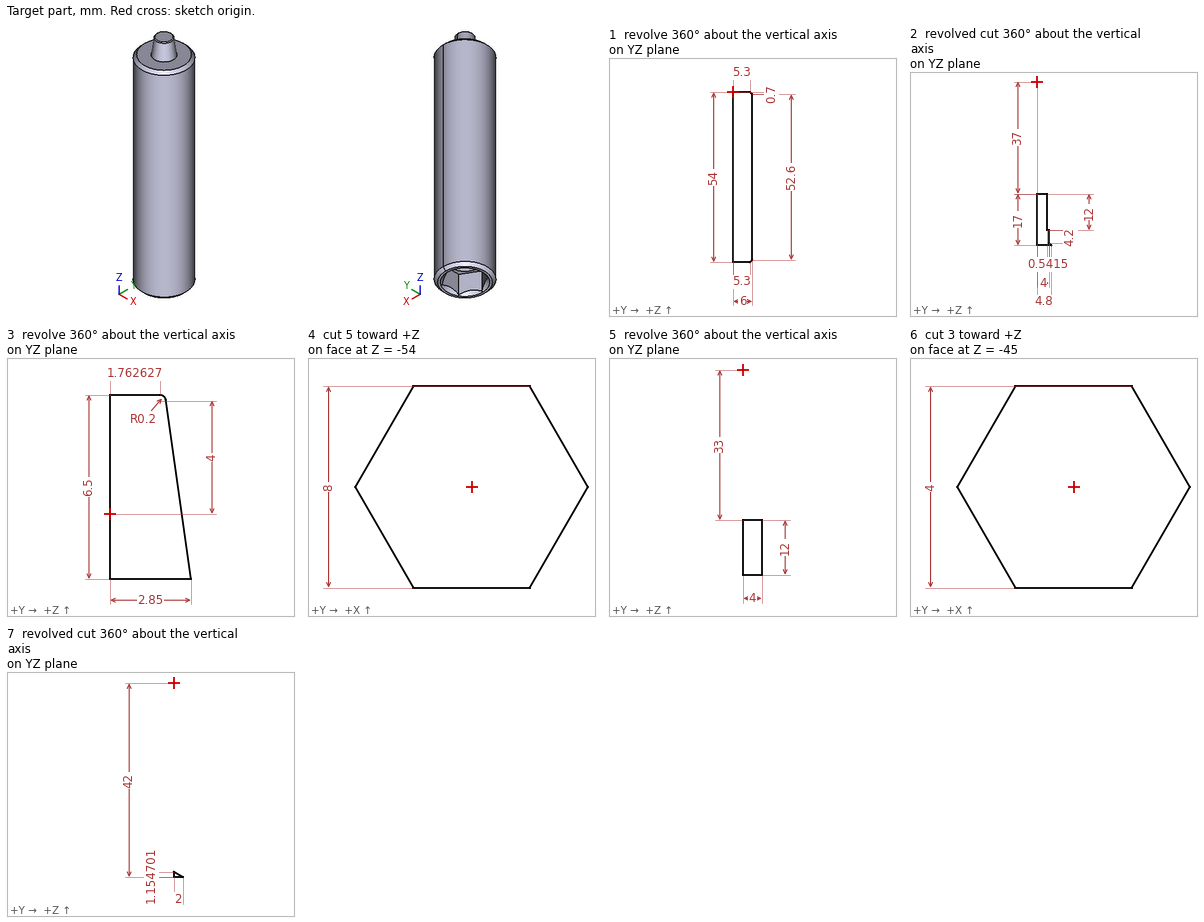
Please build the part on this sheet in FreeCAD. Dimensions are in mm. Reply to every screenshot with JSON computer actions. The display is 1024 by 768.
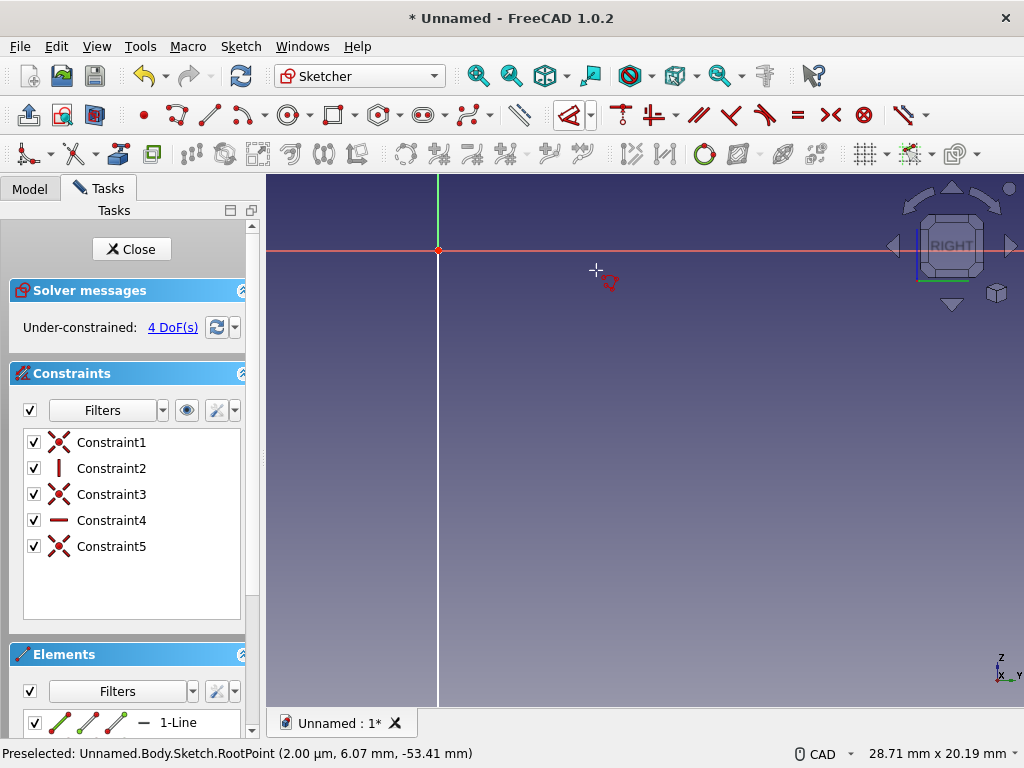
{"action": "left_click", "coordinate": [597, 269]}
{"action": "left_click", "coordinate": [578, 260]}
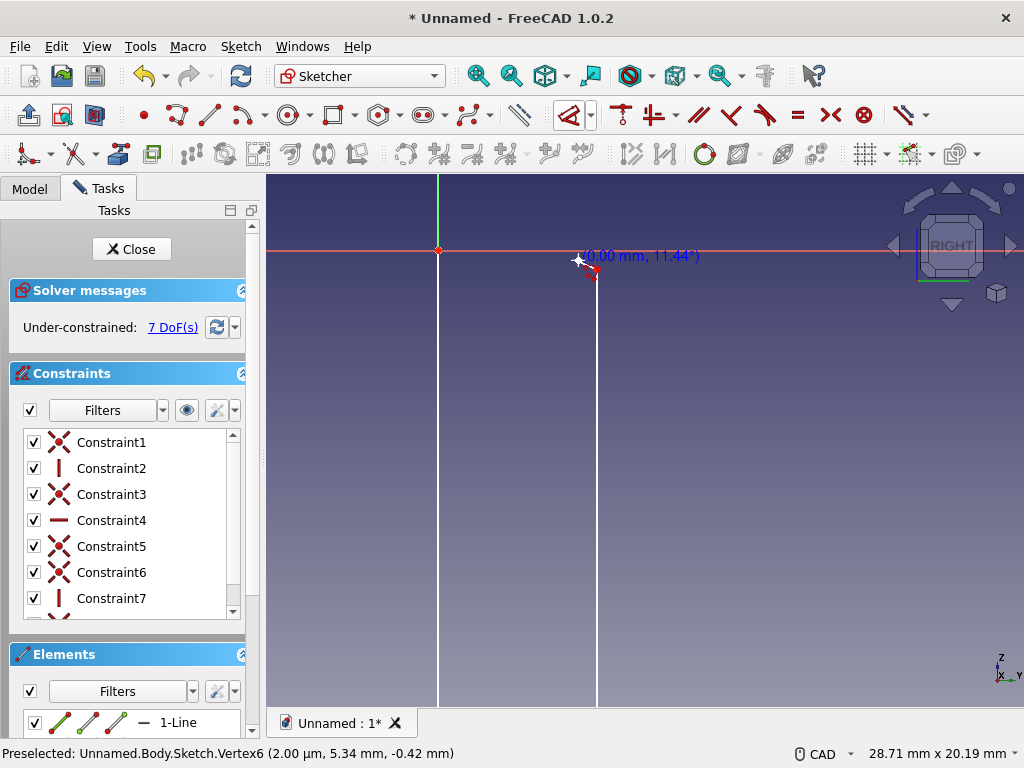
{"action": "scroll", "coordinate": [596, 269], "scroll_direction": "down", "scroll_amount": 7}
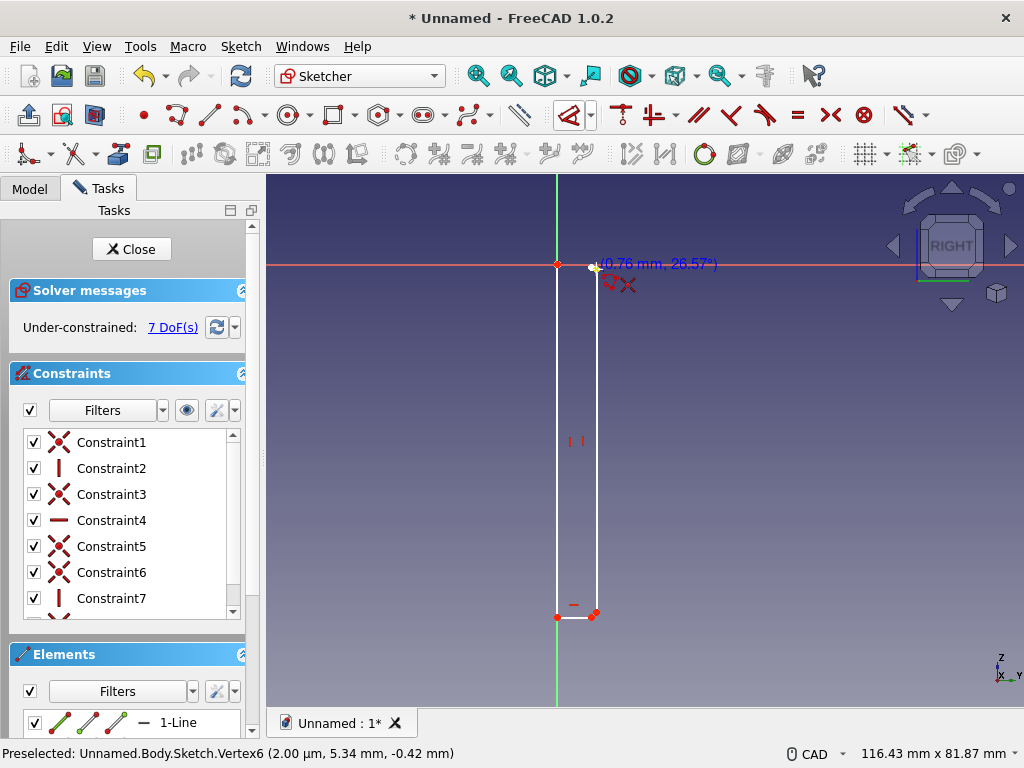
{"action": "left_click", "coordinate": [557, 265]}
{"action": "key", "text": "Escape"}
{"action": "key", "text": "Escape"}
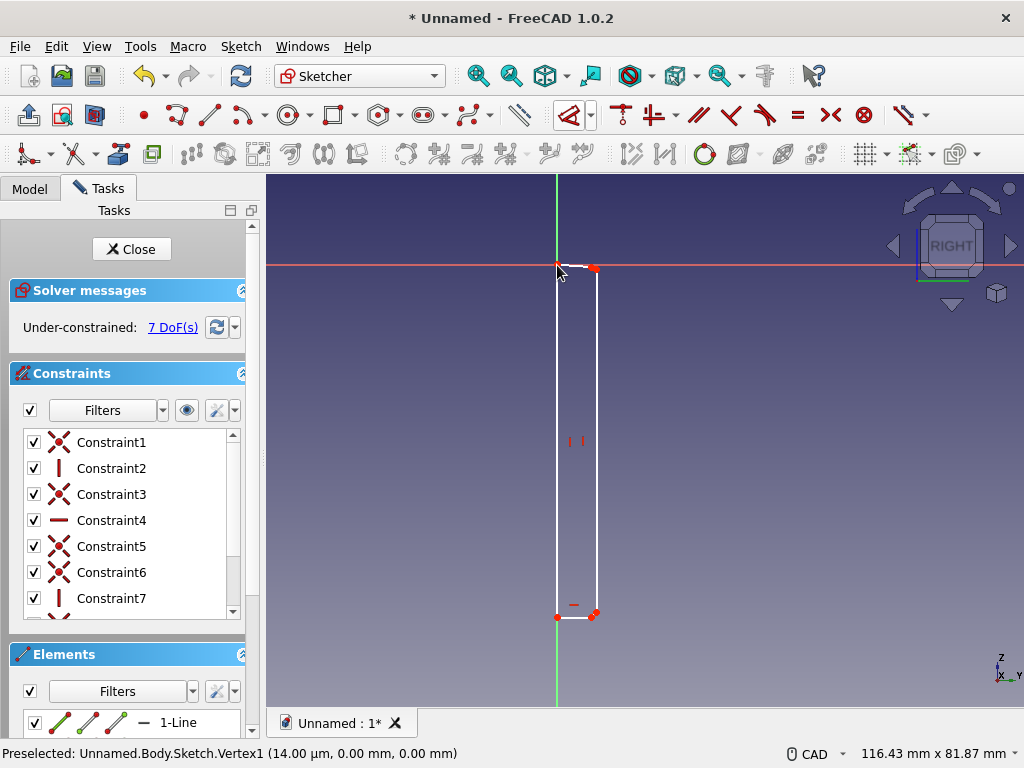
{"action": "scroll", "coordinate": [582, 266], "scroll_direction": "up", "scroll_amount": 2}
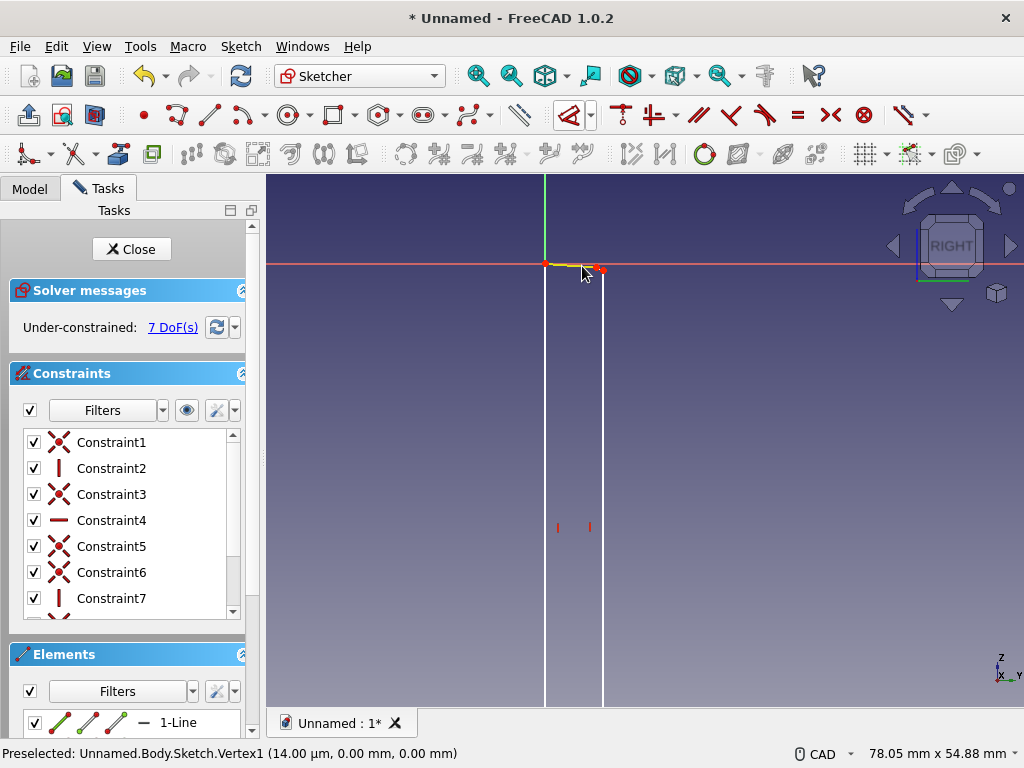
{"action": "left_click", "coordinate": [581, 267]}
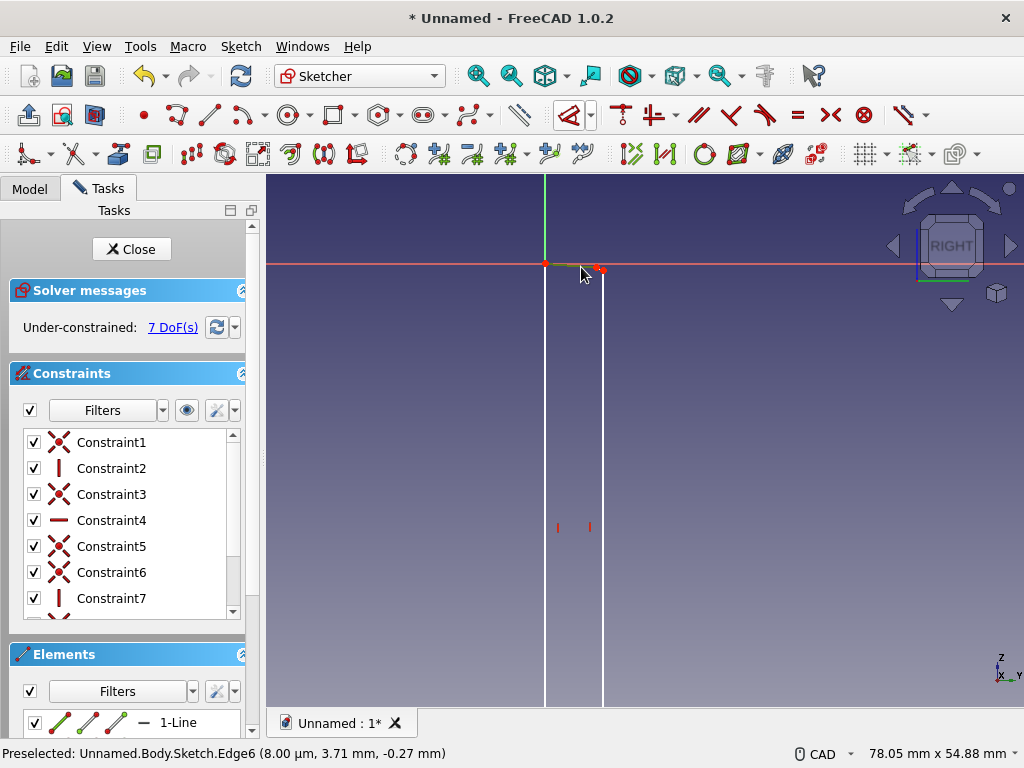
{"action": "key", "text": "h"}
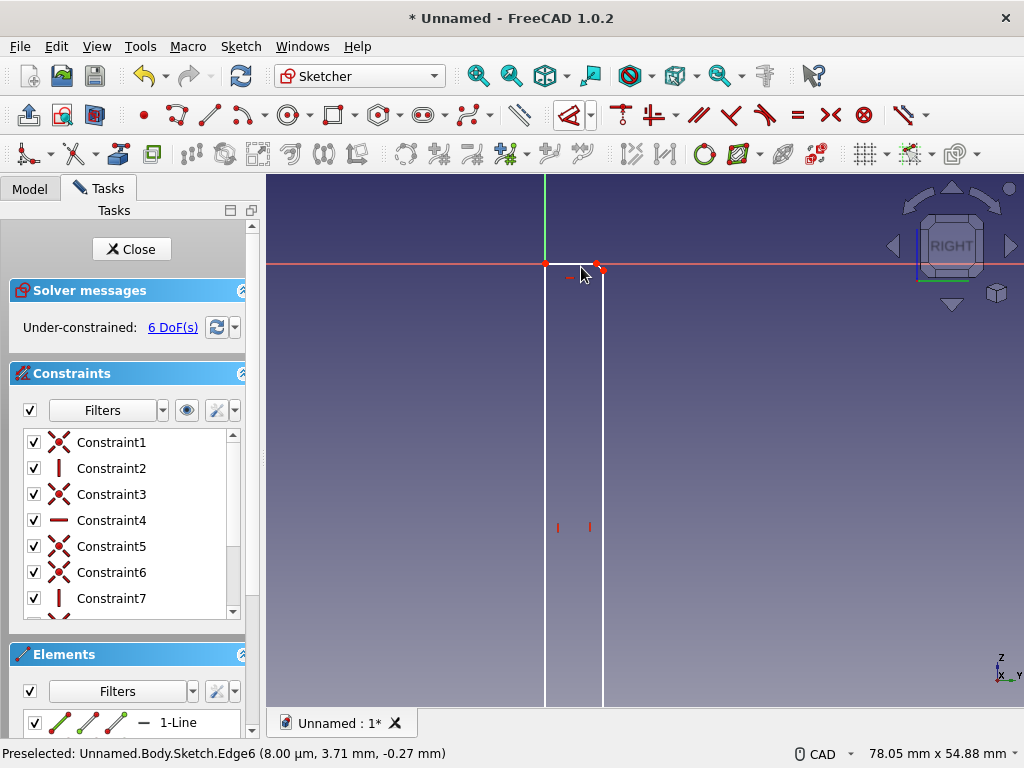
{"action": "left_click", "coordinate": [568, 116]}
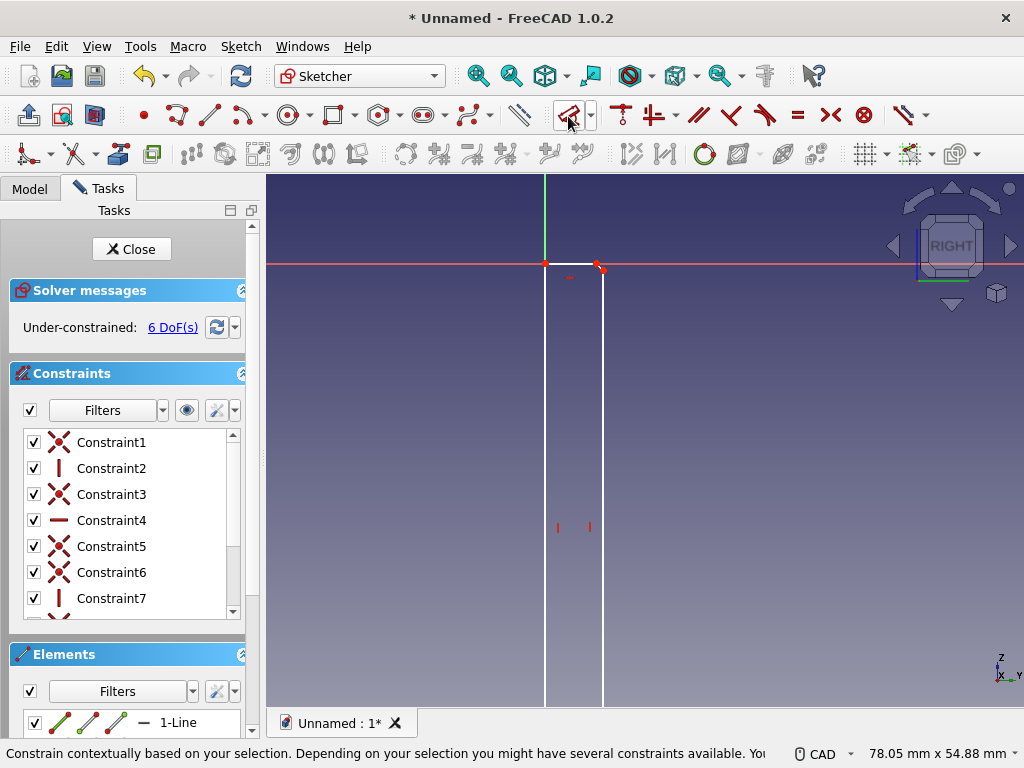
{"action": "left_click", "coordinate": [545, 422]}
{"action": "left_click", "coordinate": [511, 471]}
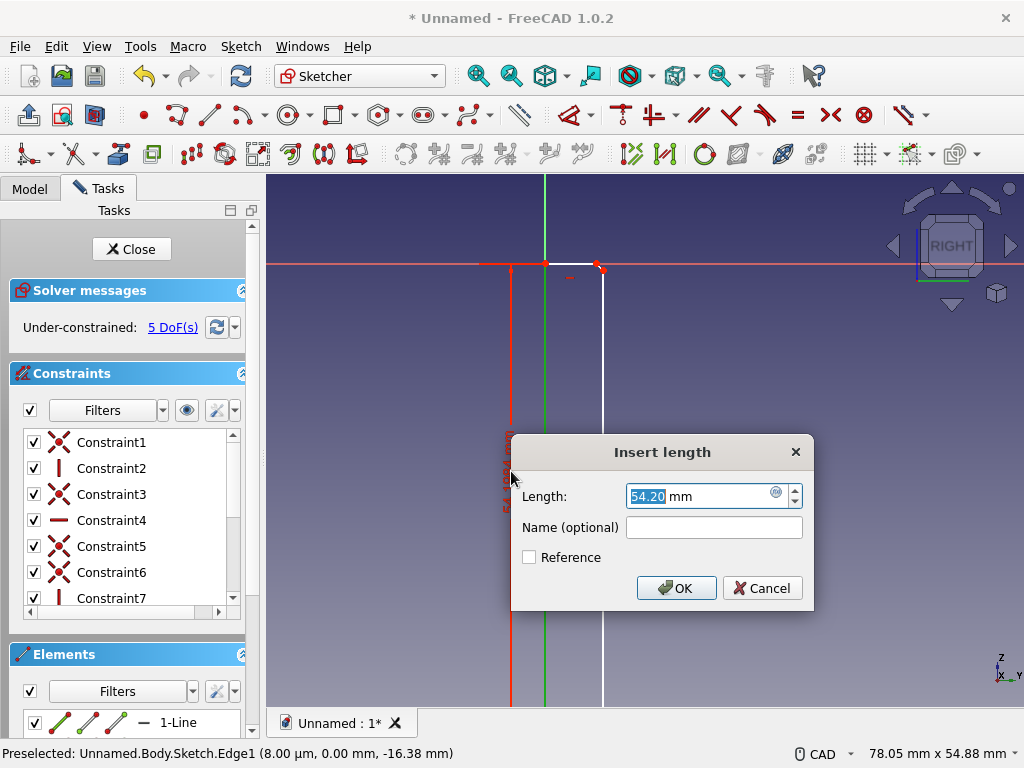
{"action": "type", "text": "54"}
{"action": "key", "text": "Return"}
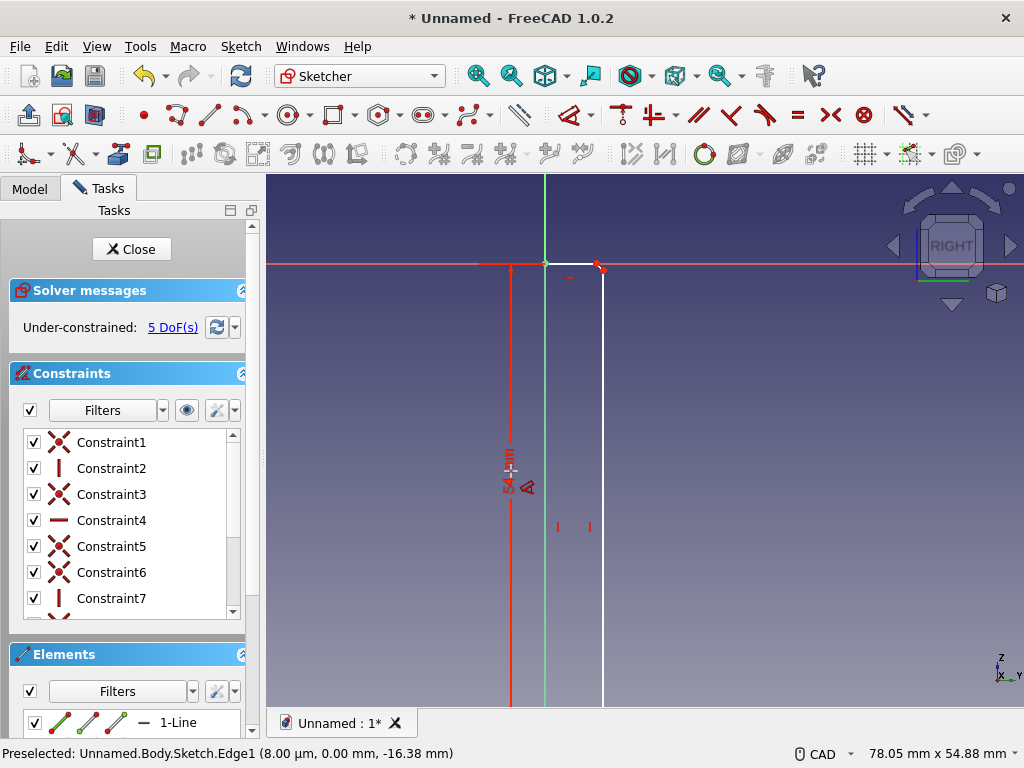
{"action": "scroll", "coordinate": [581, 266], "scroll_direction": "down", "scroll_amount": 2}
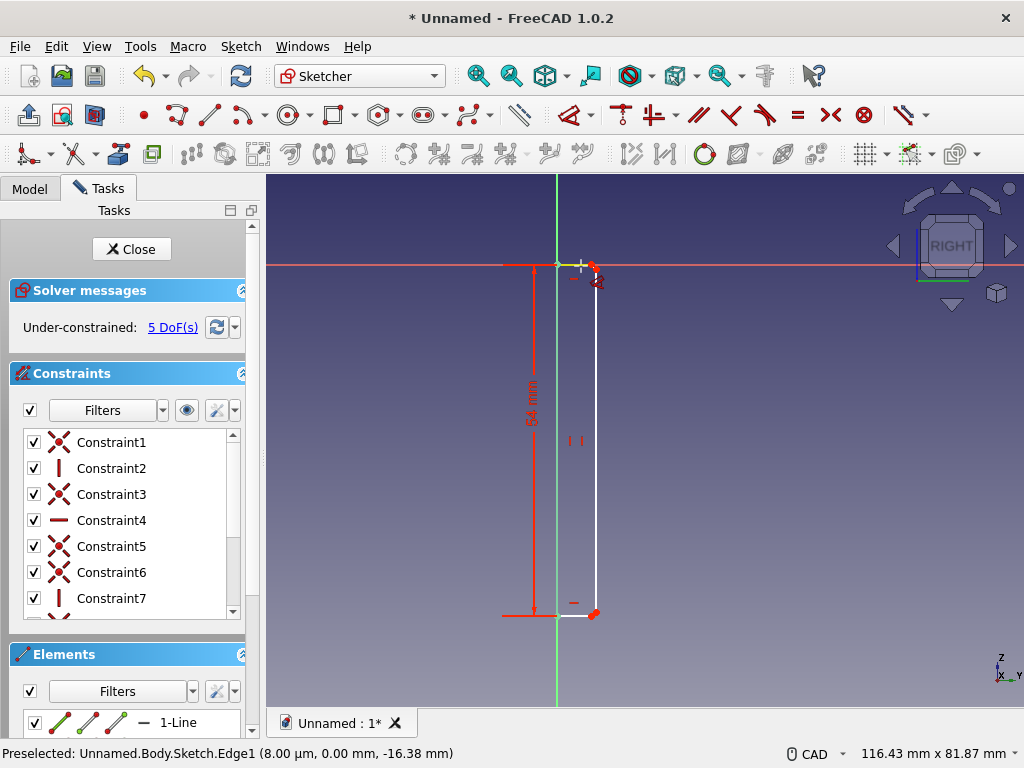
{"action": "scroll", "coordinate": [596, 612], "scroll_direction": "up", "scroll_amount": 4}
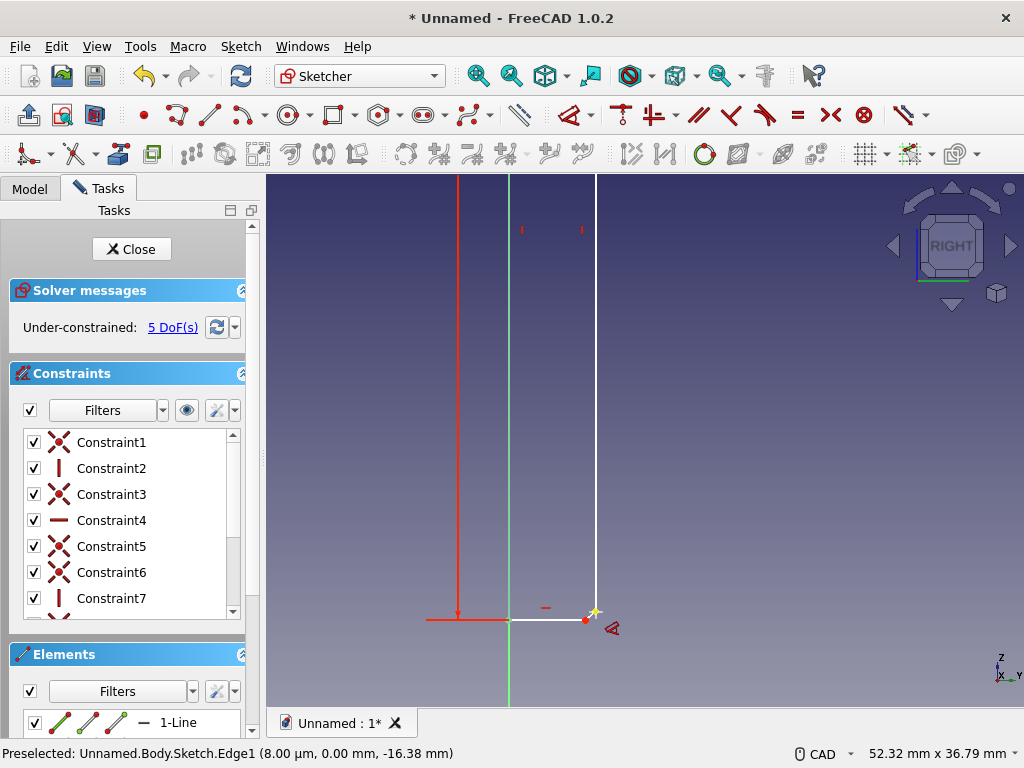
{"action": "left_click", "coordinate": [596, 611]}
{"action": "left_click", "coordinate": [552, 645]}